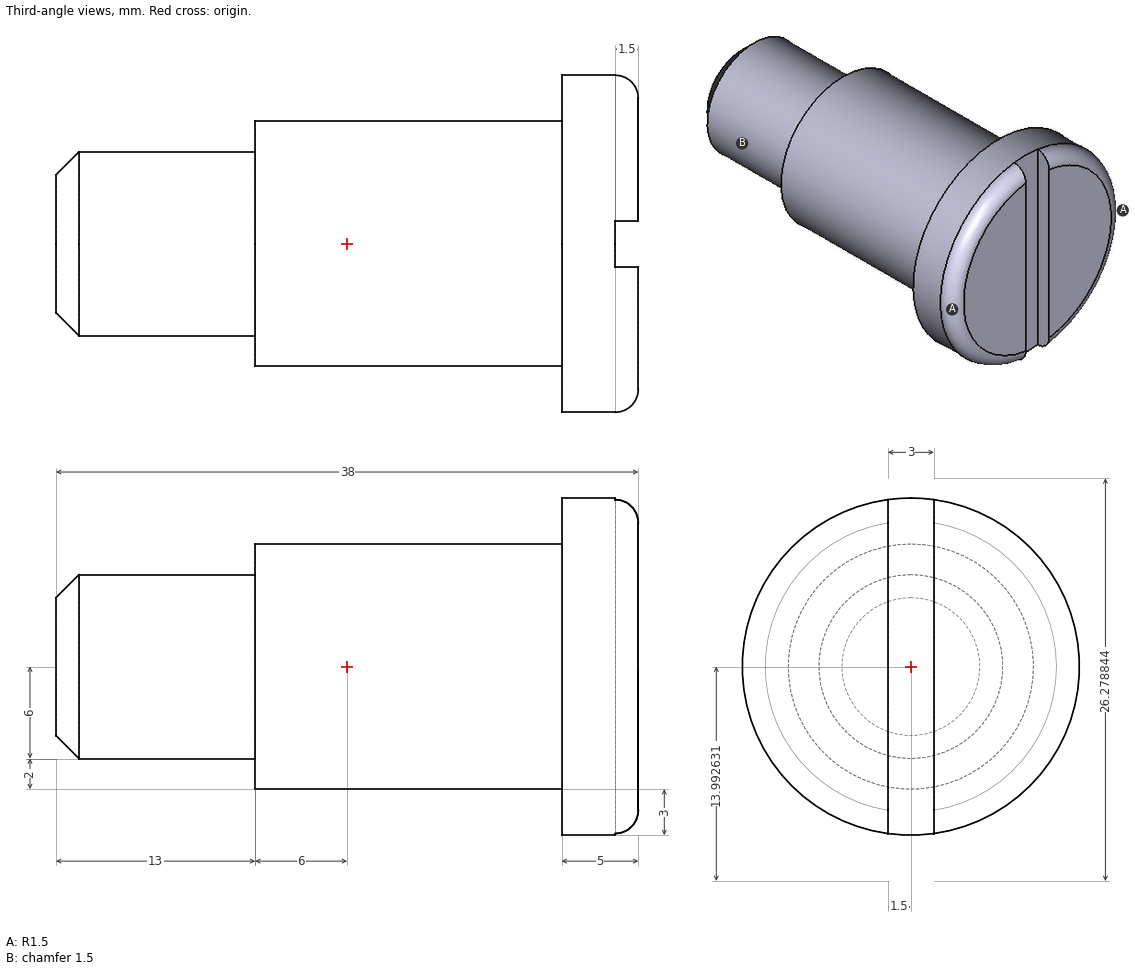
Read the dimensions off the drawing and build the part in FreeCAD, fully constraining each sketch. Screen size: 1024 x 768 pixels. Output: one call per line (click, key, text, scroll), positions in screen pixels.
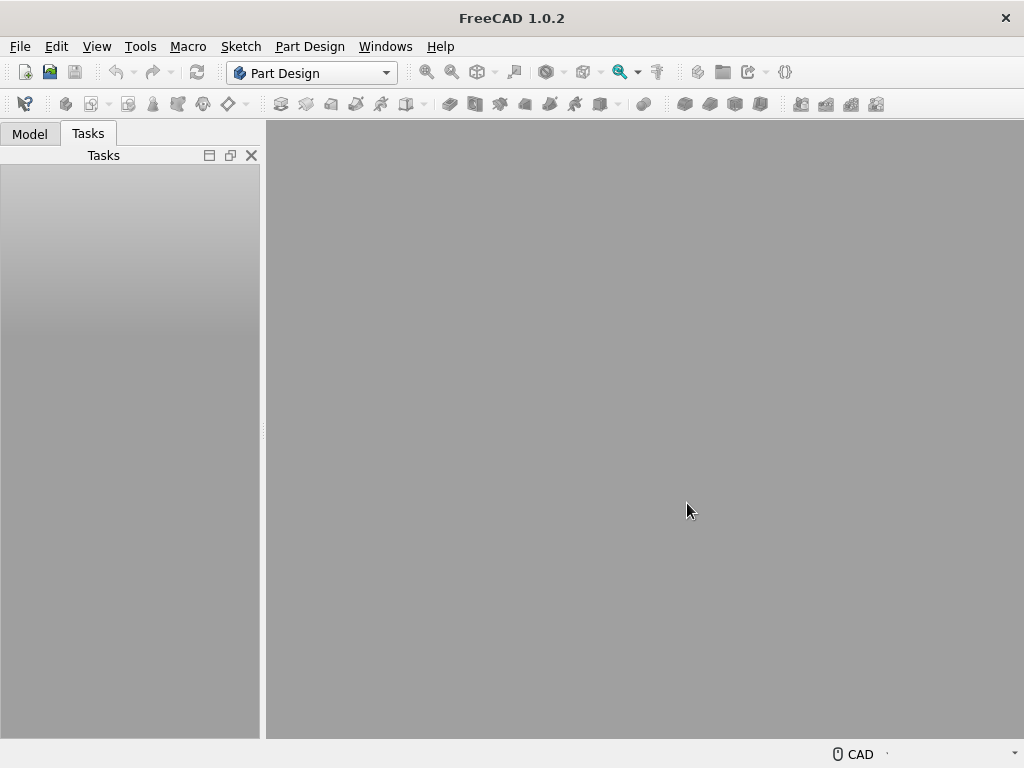
click(25, 72)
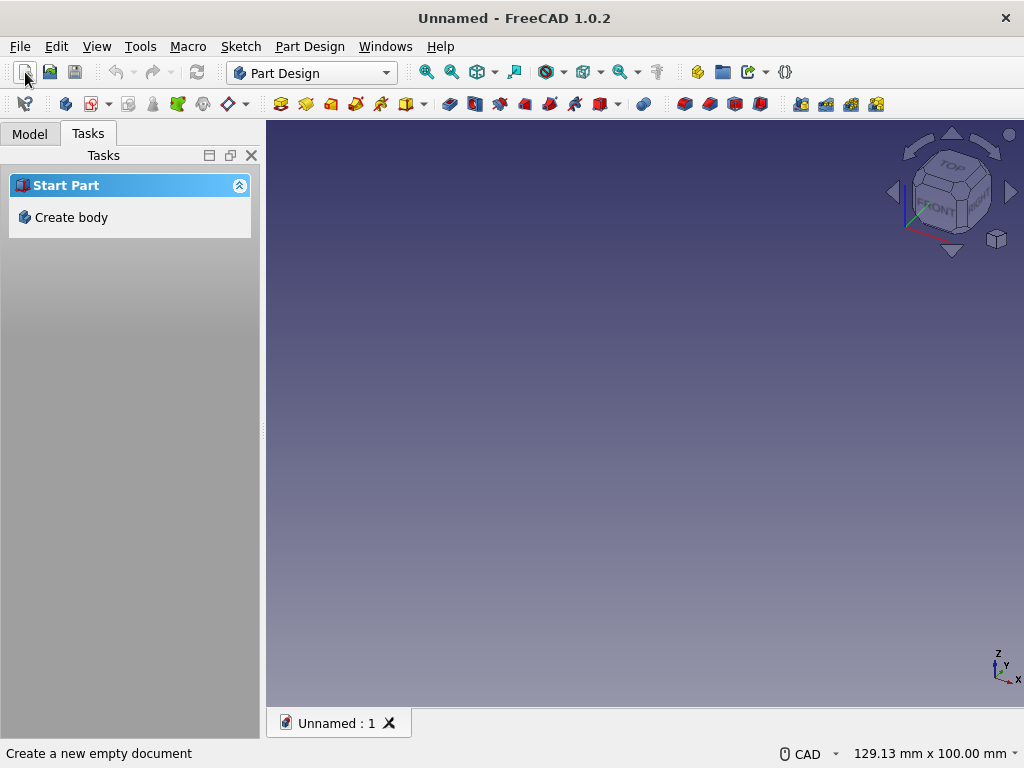
click(90, 104)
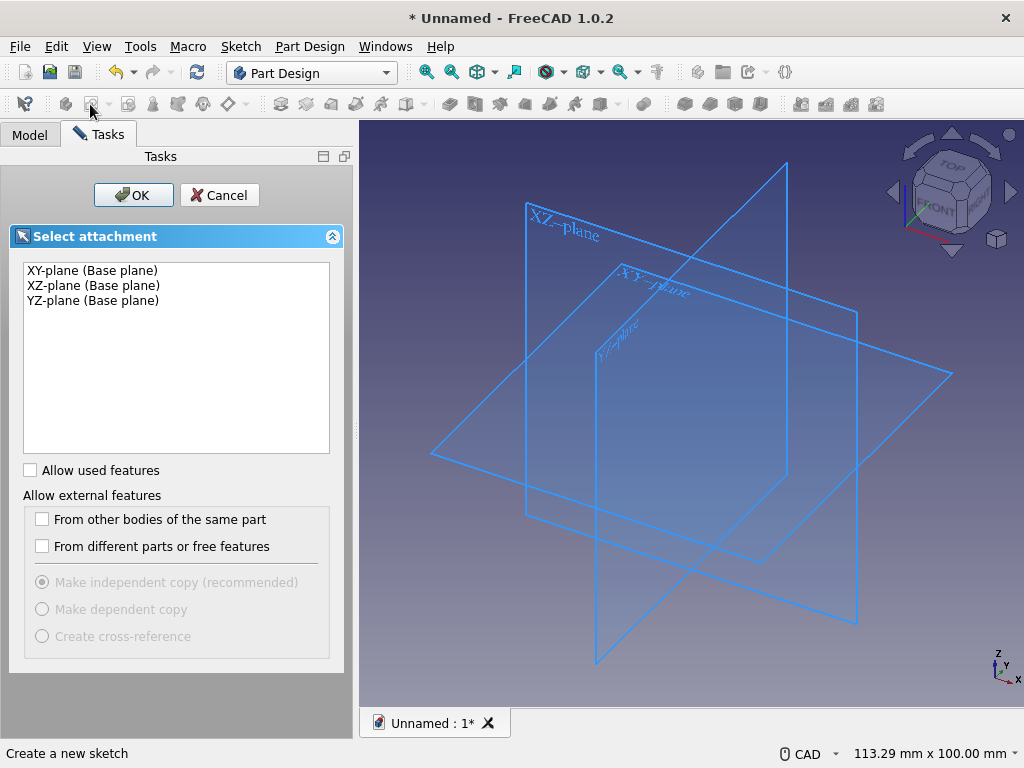
click(84, 286)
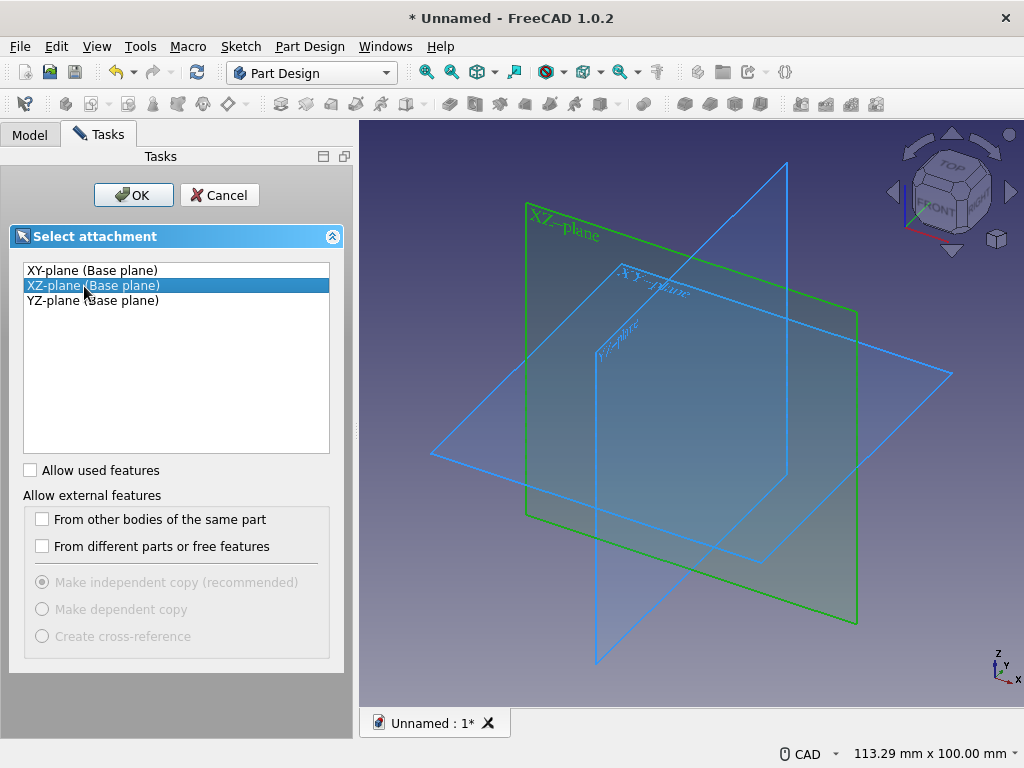
click(134, 195)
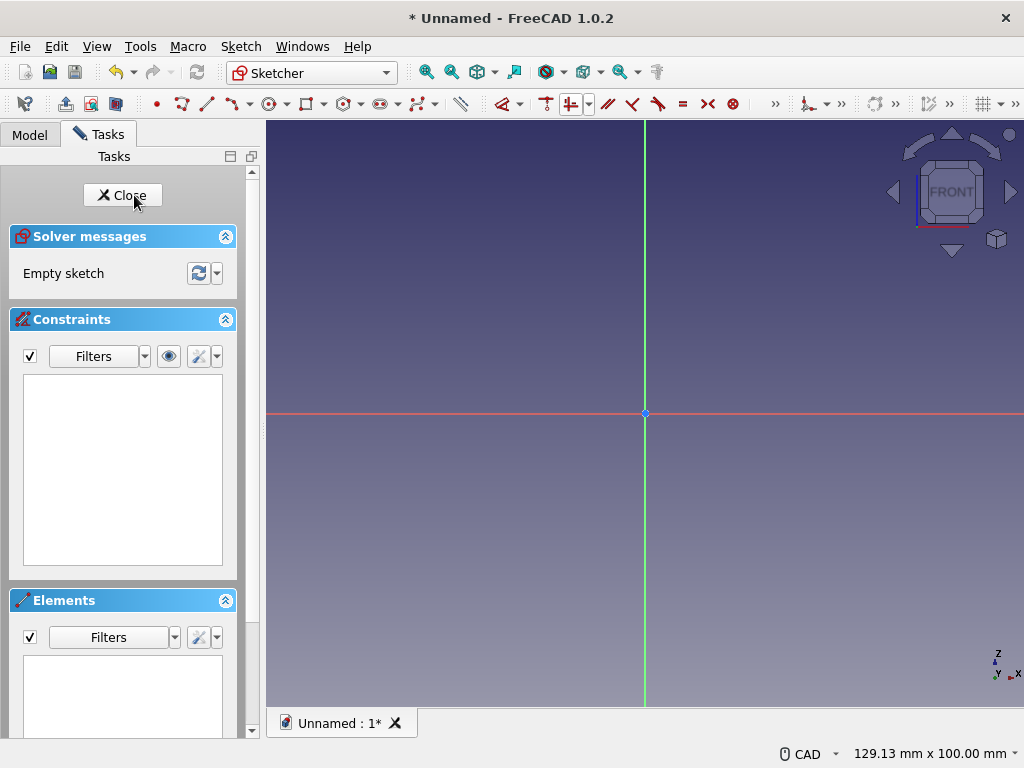
scroll(728, 485, up, 3)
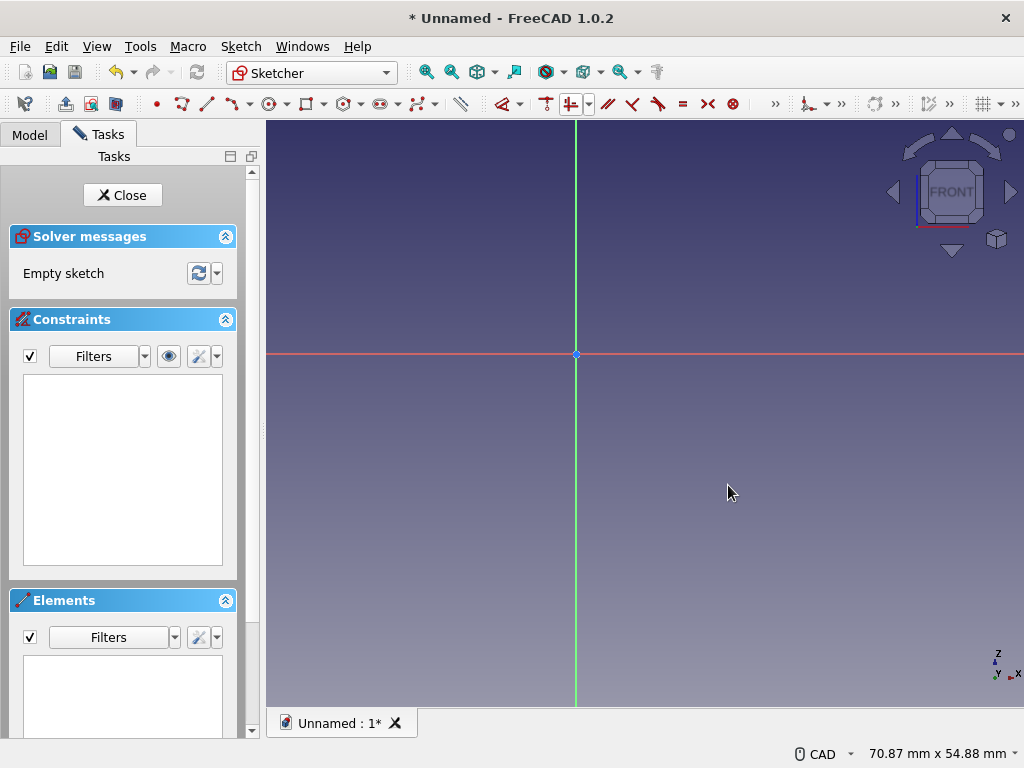
click(182, 104)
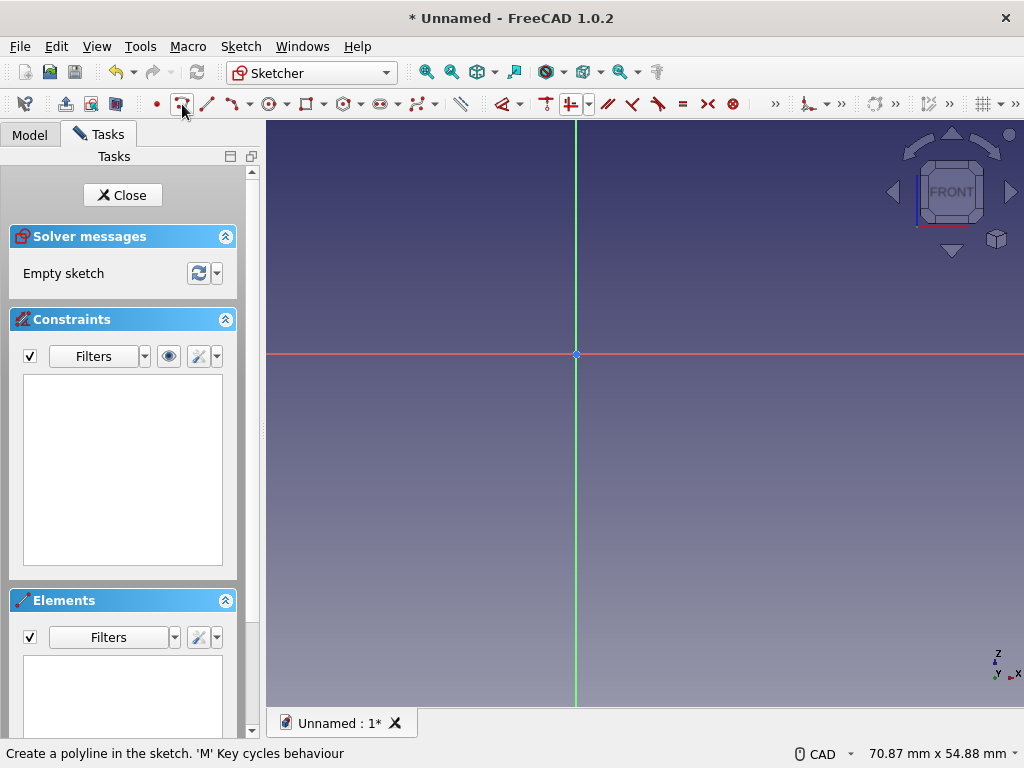
click(512, 418)
click(373, 418)
click(373, 354)
click(779, 363)
click(779, 472)
click(726, 472)
click(726, 440)
click(512, 440)
click(512, 419)
key(Escape)
key(Escape)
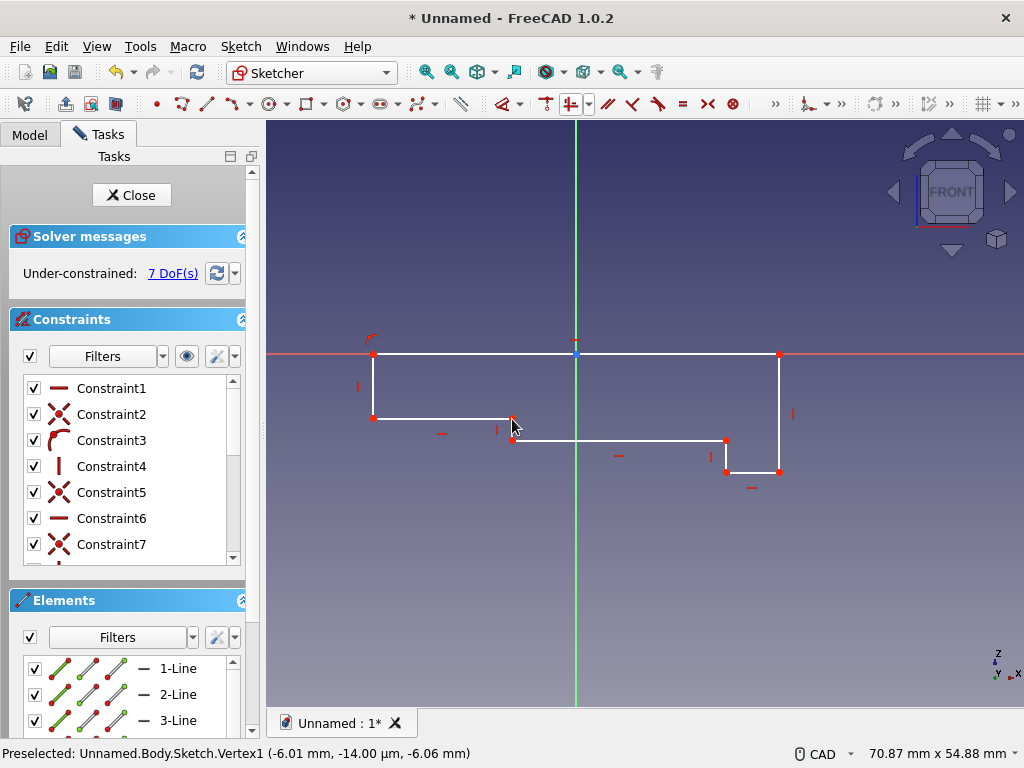
key(d)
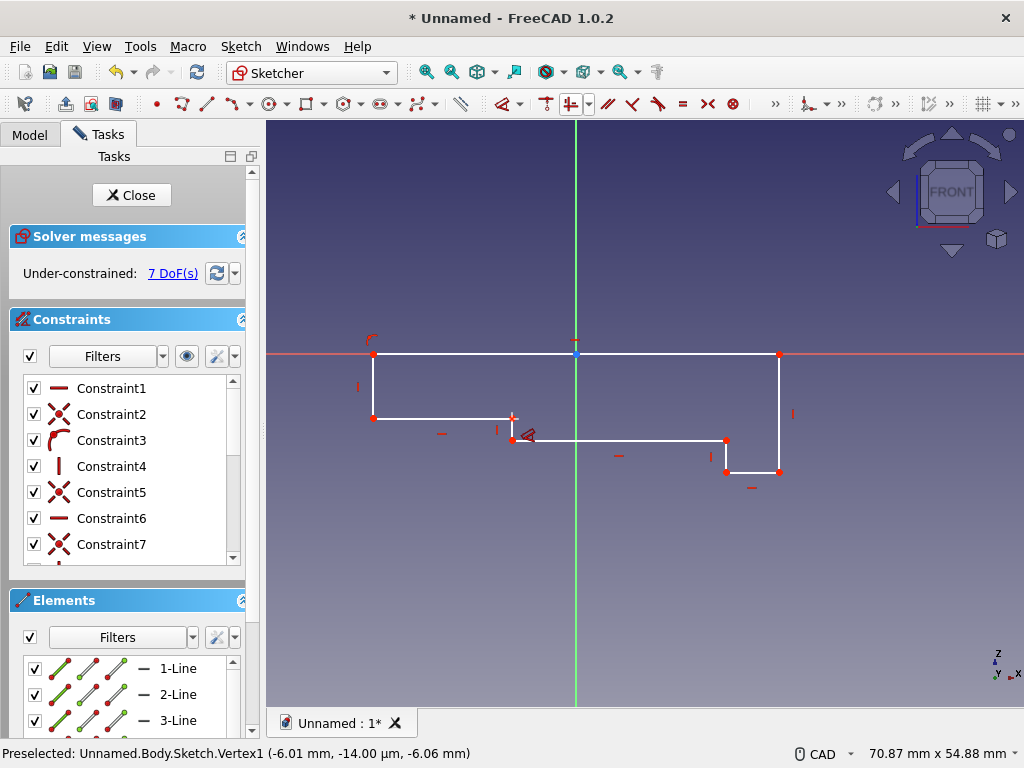
click(373, 400)
click(339, 387)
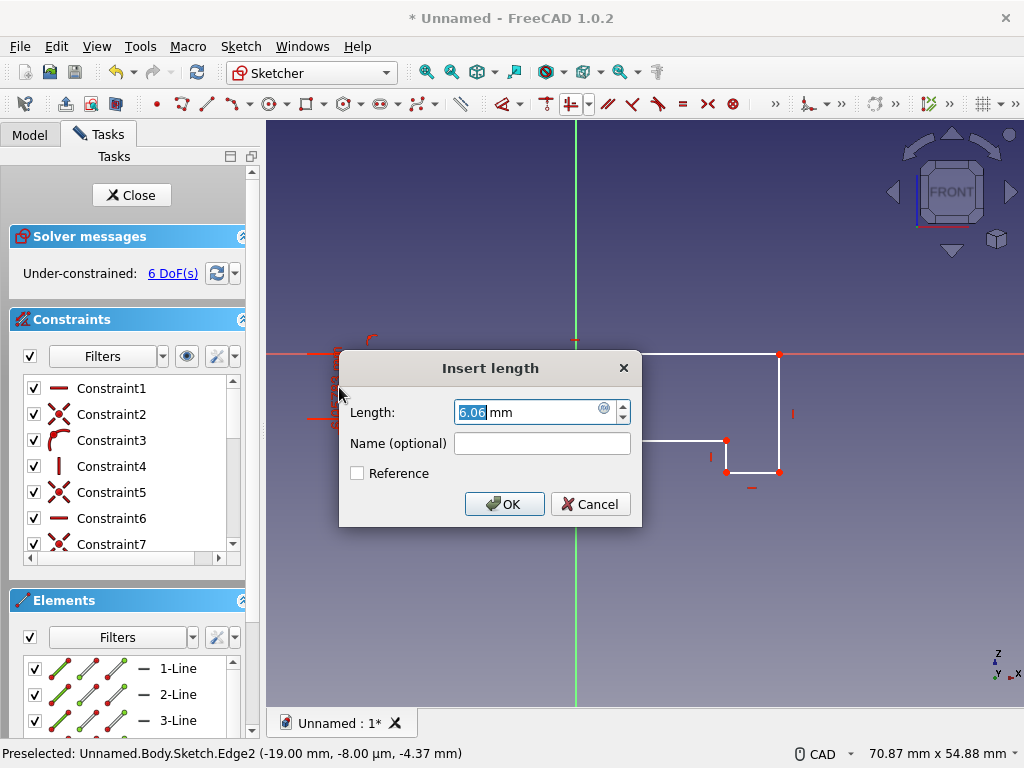
text(6)
key(Return)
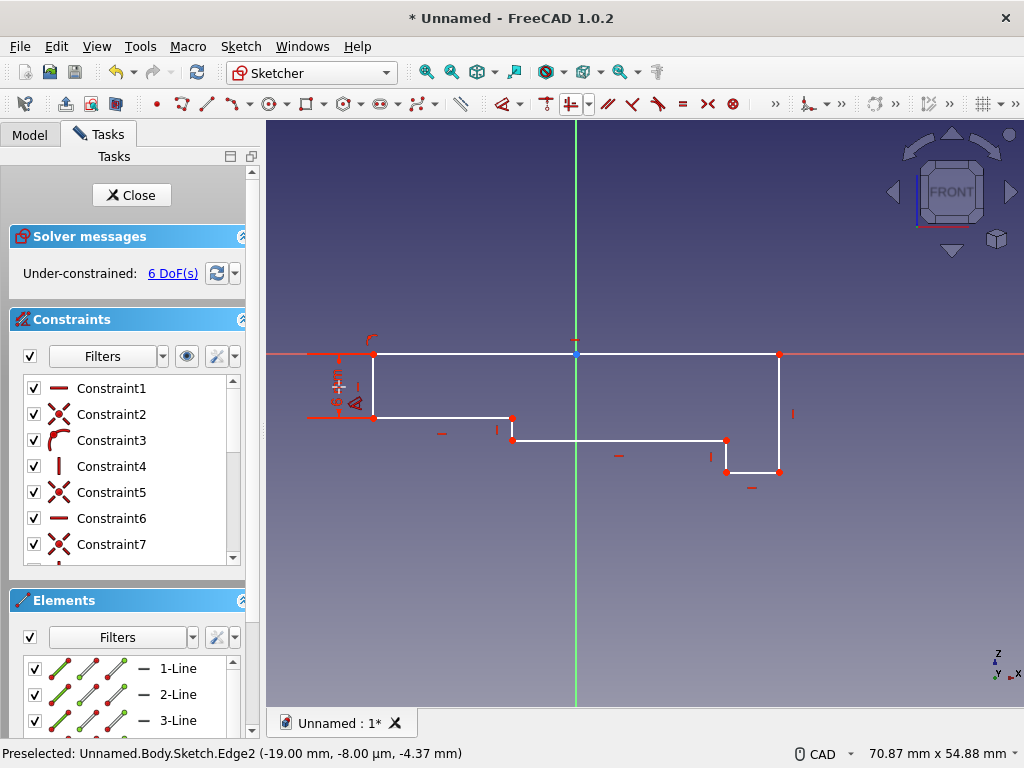
click(763, 473)
click(752, 507)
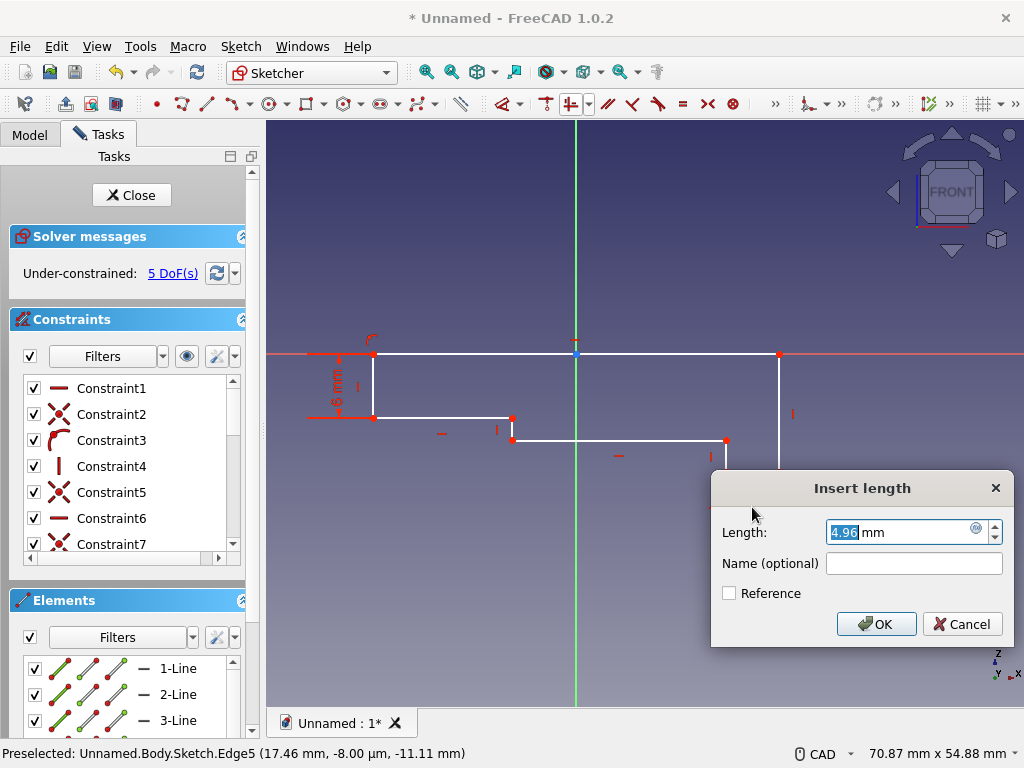
text(5)
key(Return)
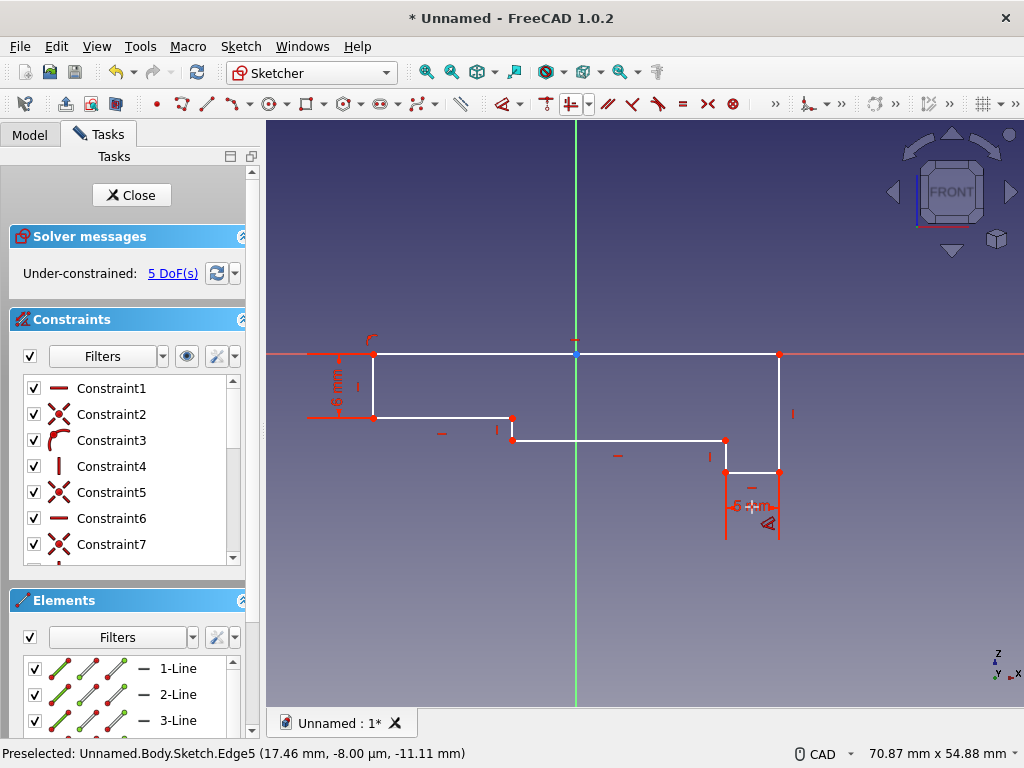
scroll(726, 463, up, 2)